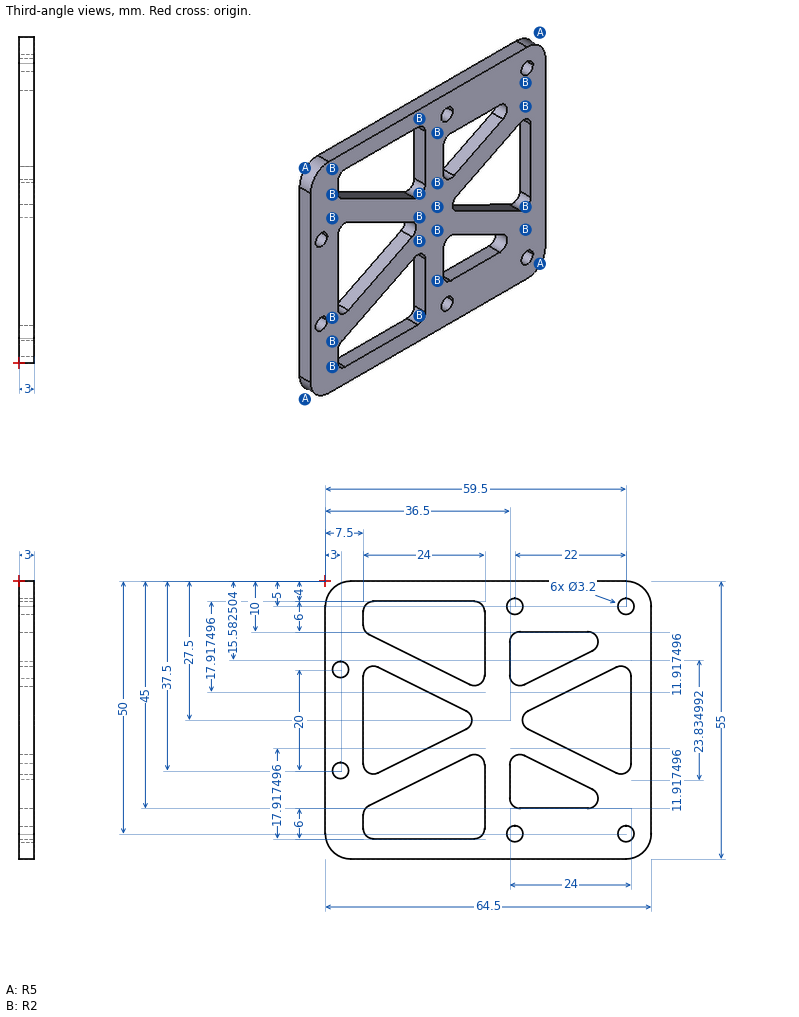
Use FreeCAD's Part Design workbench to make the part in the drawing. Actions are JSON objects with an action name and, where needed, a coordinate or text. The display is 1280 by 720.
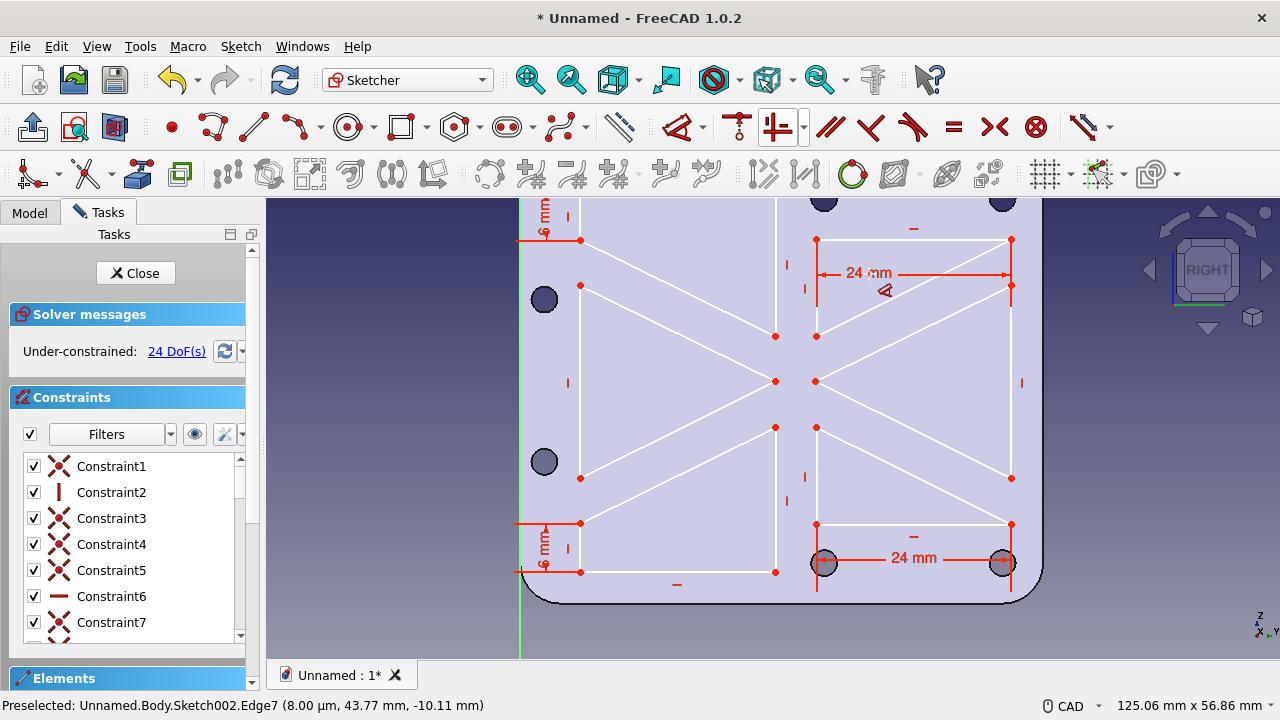
{"action": "scroll", "coordinate": [581, 559], "scroll_direction": "down", "scroll_amount": 2}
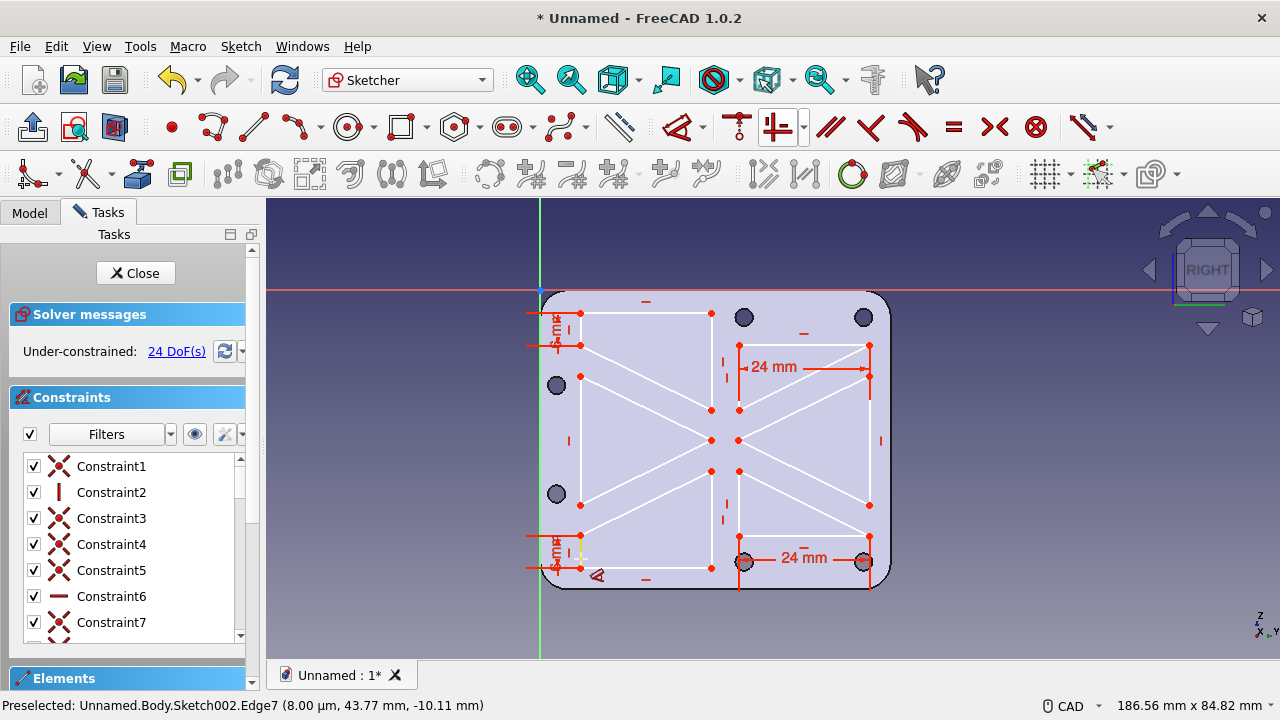
{"action": "left_click", "coordinate": [620, 313]}
{"action": "left_click", "coordinate": [646, 347]}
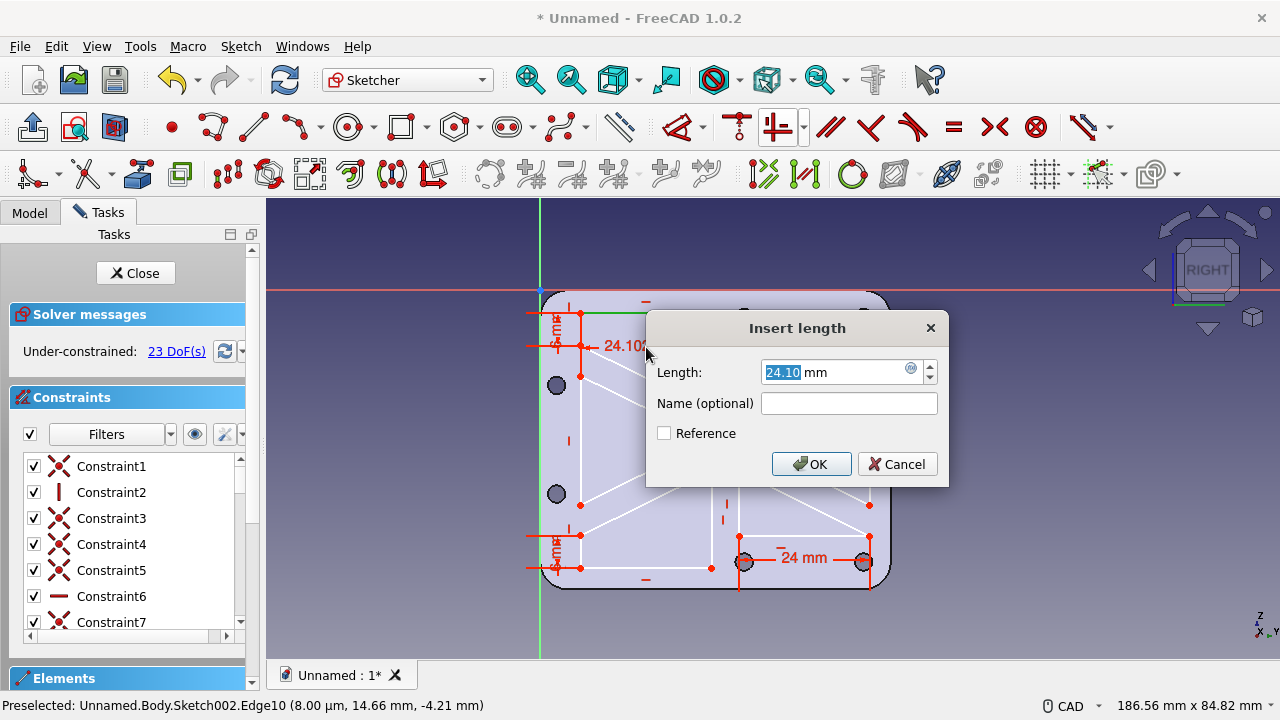
{"action": "type", "text": "24"}
{"action": "key", "text": "Return"}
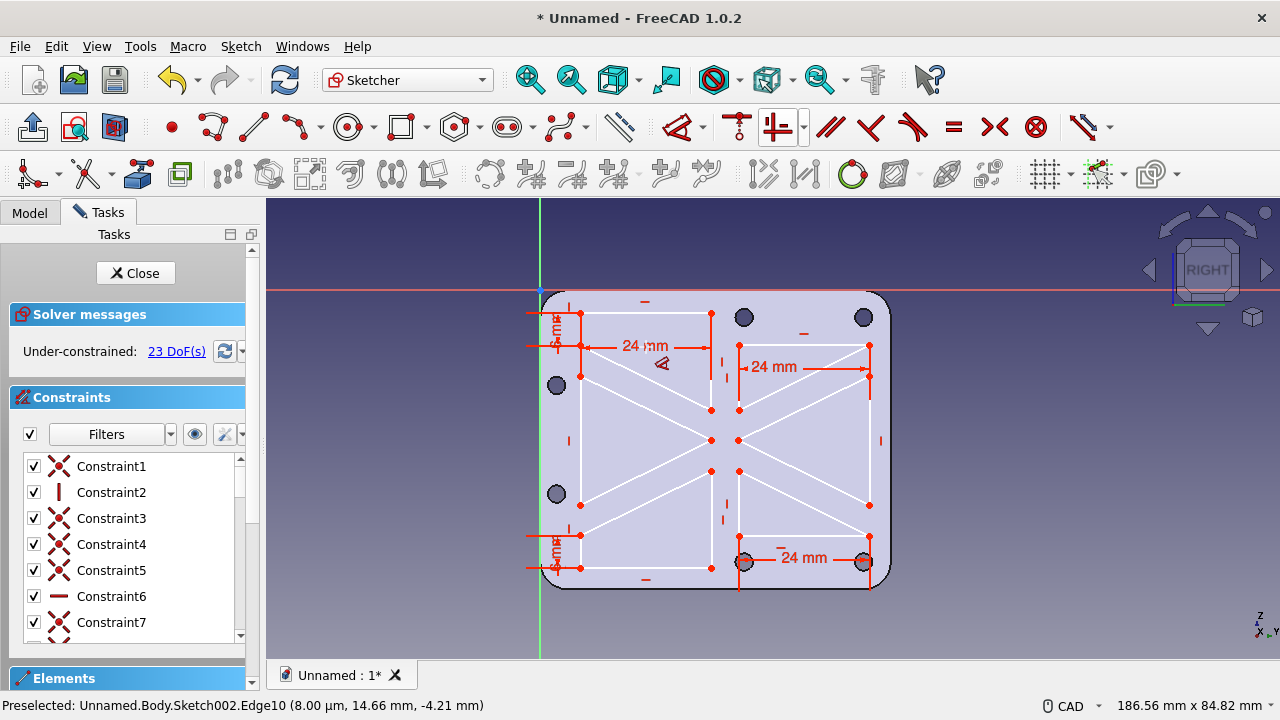
{"action": "left_click", "coordinate": [672, 568]}
{"action": "left_click", "coordinate": [646, 602]}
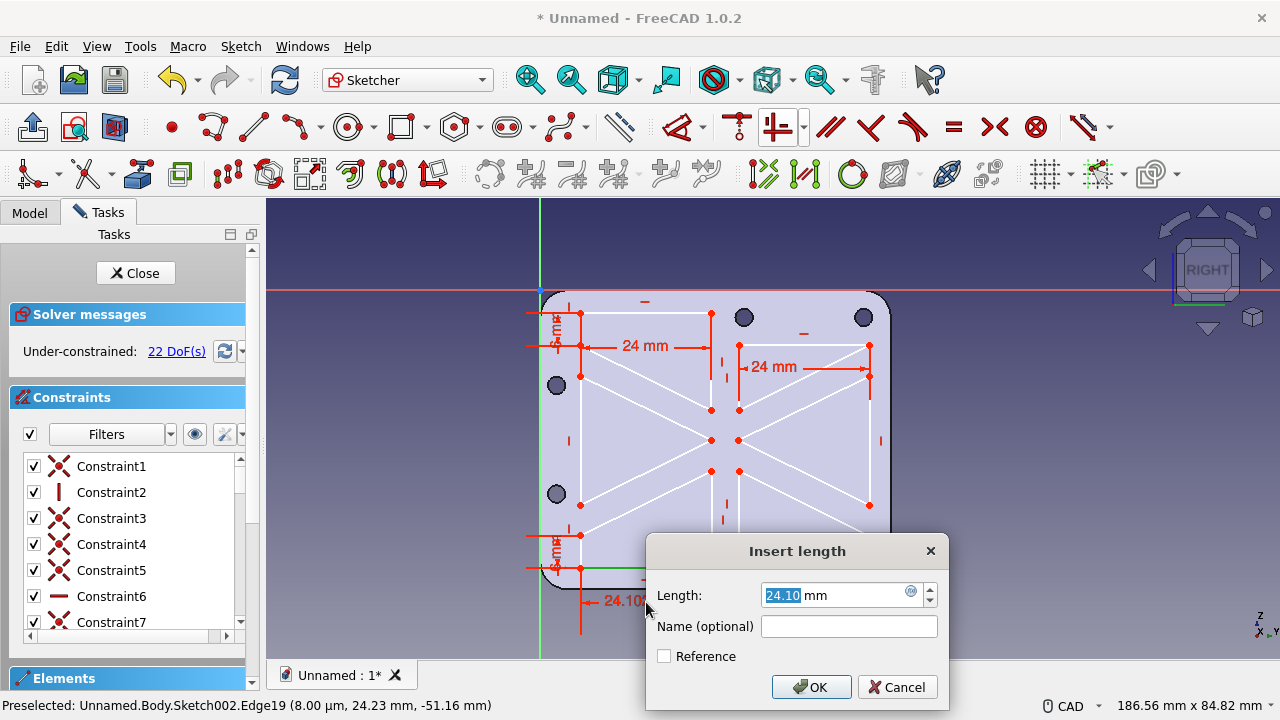
{"action": "type", "text": "24"}
{"action": "key", "text": "Return"}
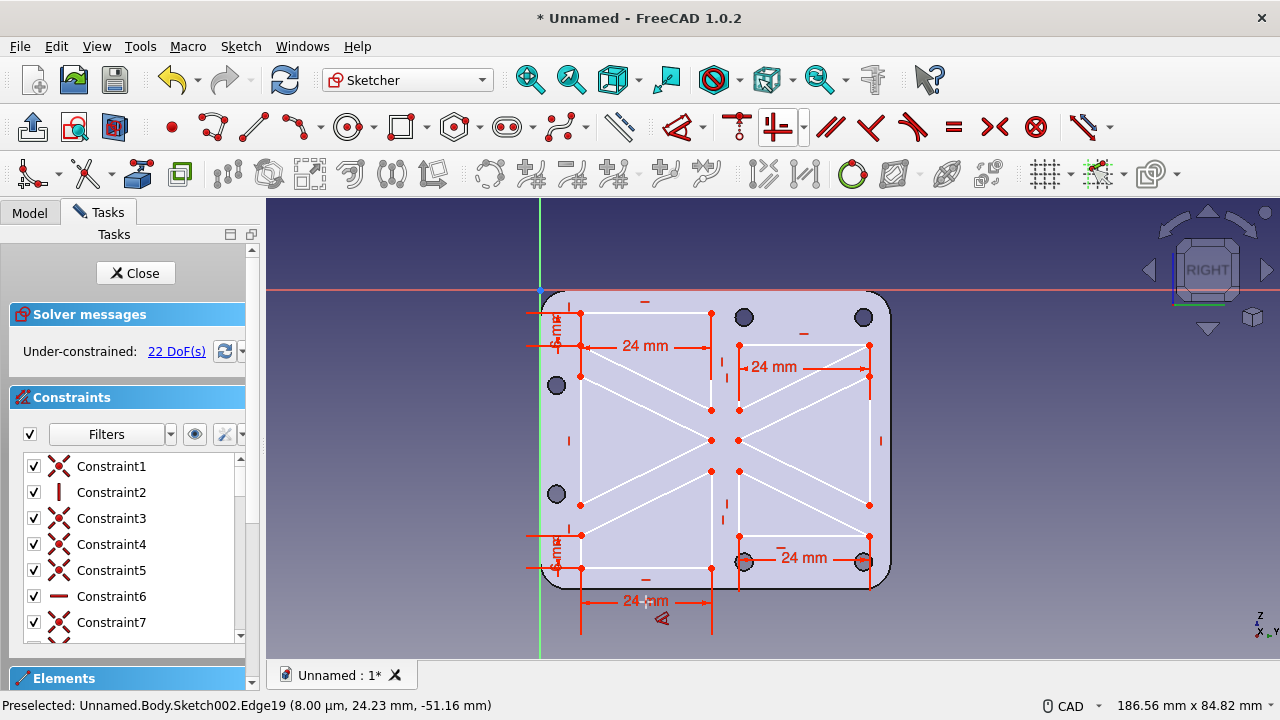
{"action": "scroll", "coordinate": [581, 313], "scroll_direction": "up", "scroll_amount": 4}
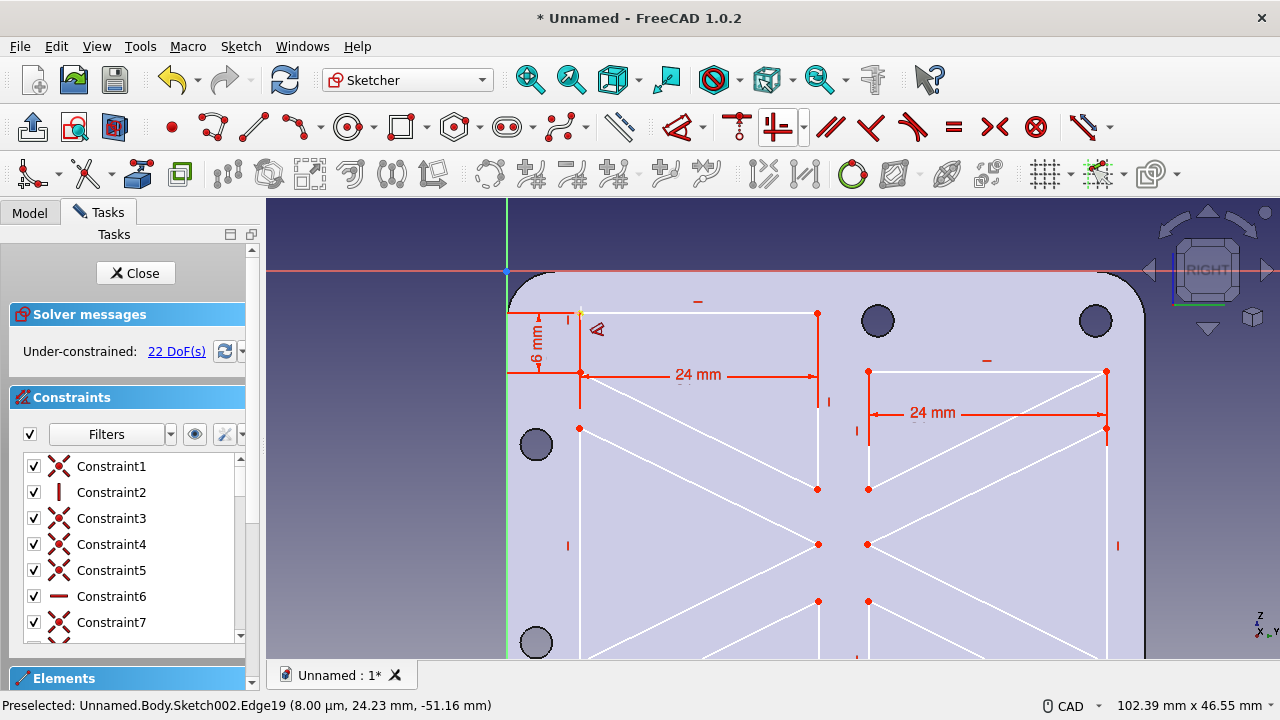
{"action": "left_click", "coordinate": [580, 313]}
{"action": "left_click", "coordinate": [456, 288]}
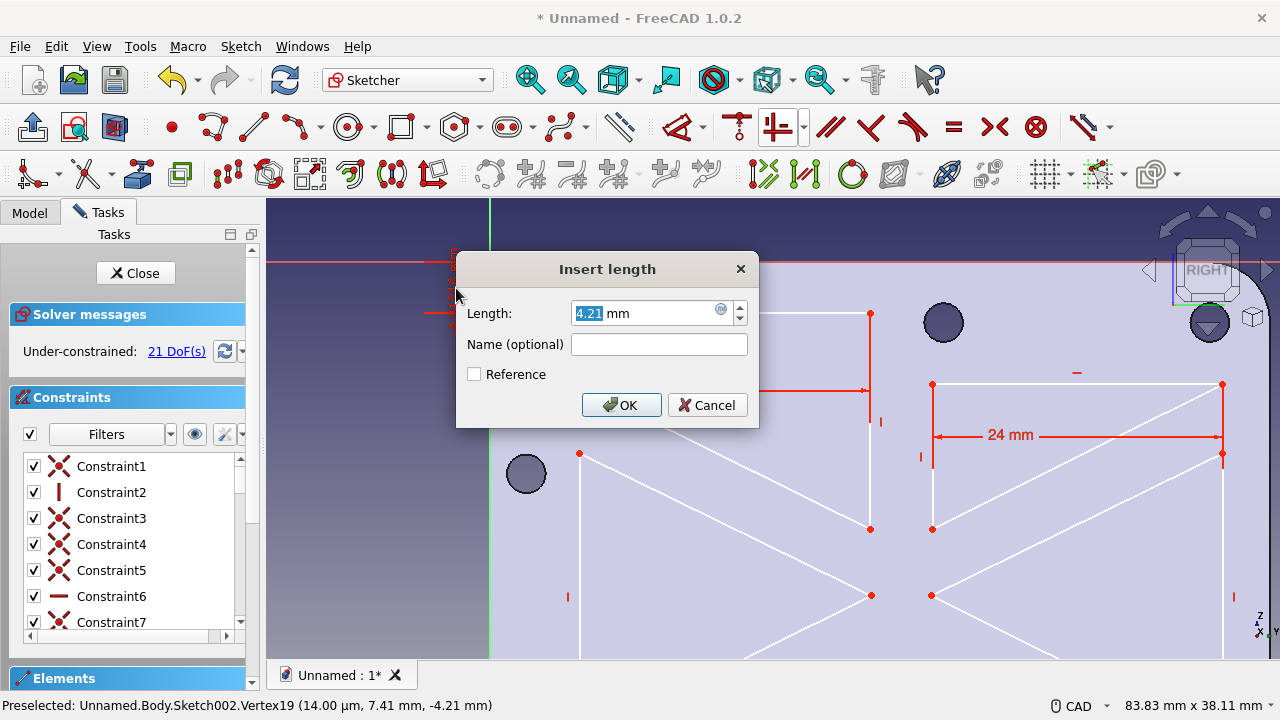
{"action": "type", "text": "4"}
{"action": "key", "text": "Return"}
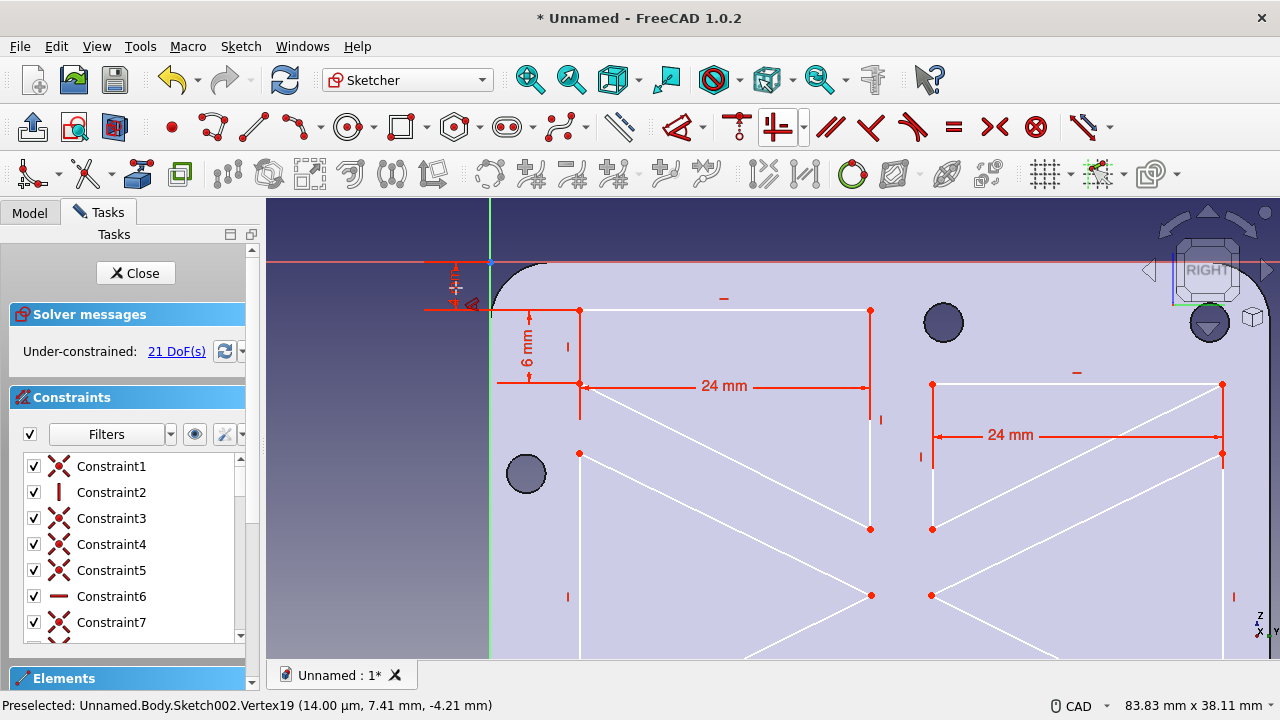
{"action": "scroll", "coordinate": [581, 313], "scroll_direction": "down", "scroll_amount": 4}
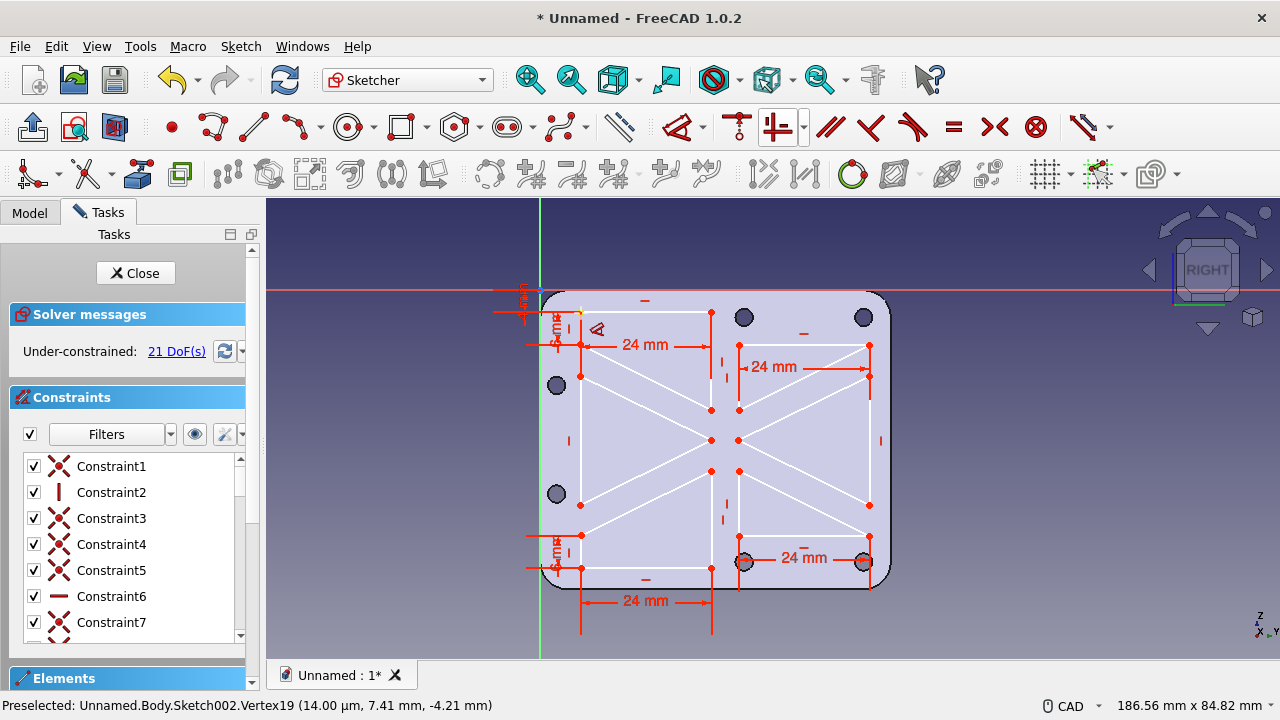
{"action": "left_click", "coordinate": [870, 536]}
{"action": "left_click", "coordinate": [904, 413]}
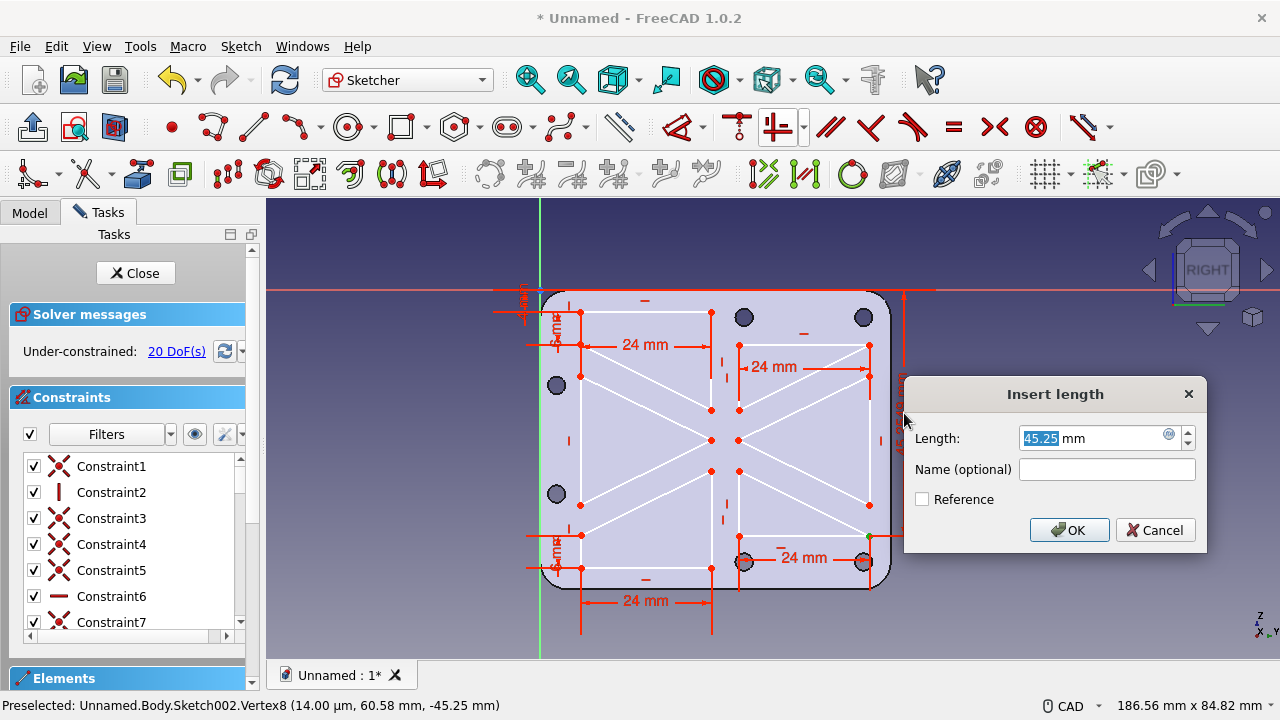
{"action": "type", "text": "45"}
{"action": "key", "text": "Return"}